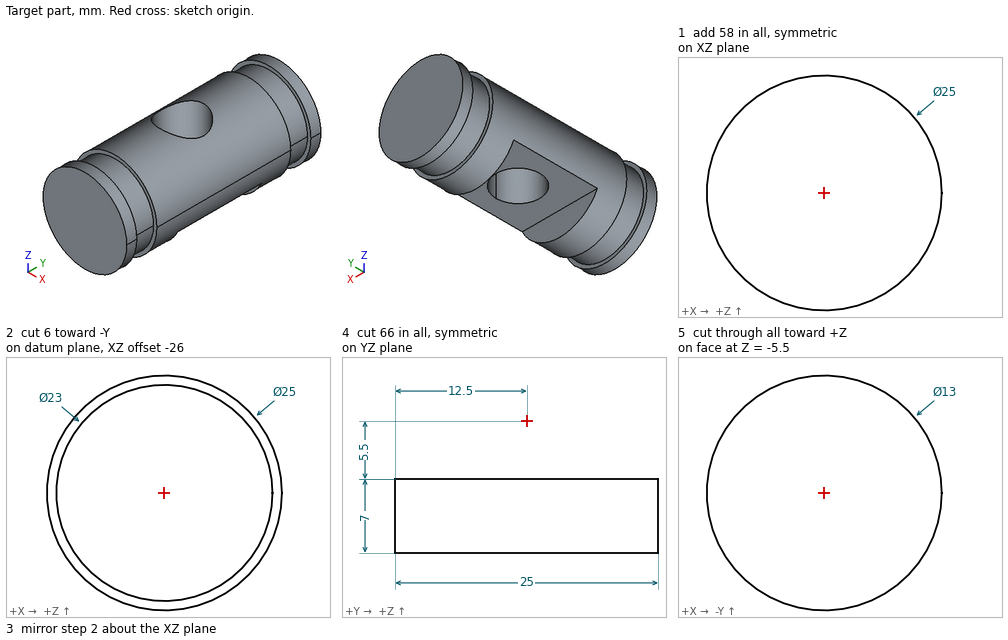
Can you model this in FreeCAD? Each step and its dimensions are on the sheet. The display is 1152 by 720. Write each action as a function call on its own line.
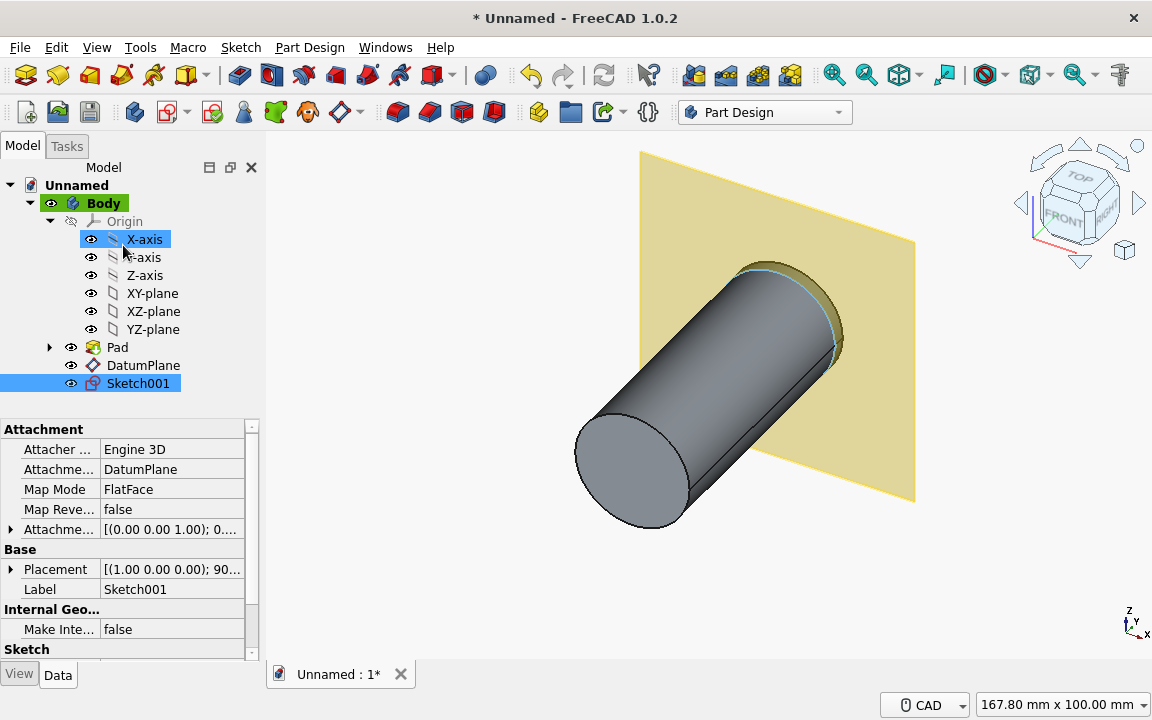
click(240, 76)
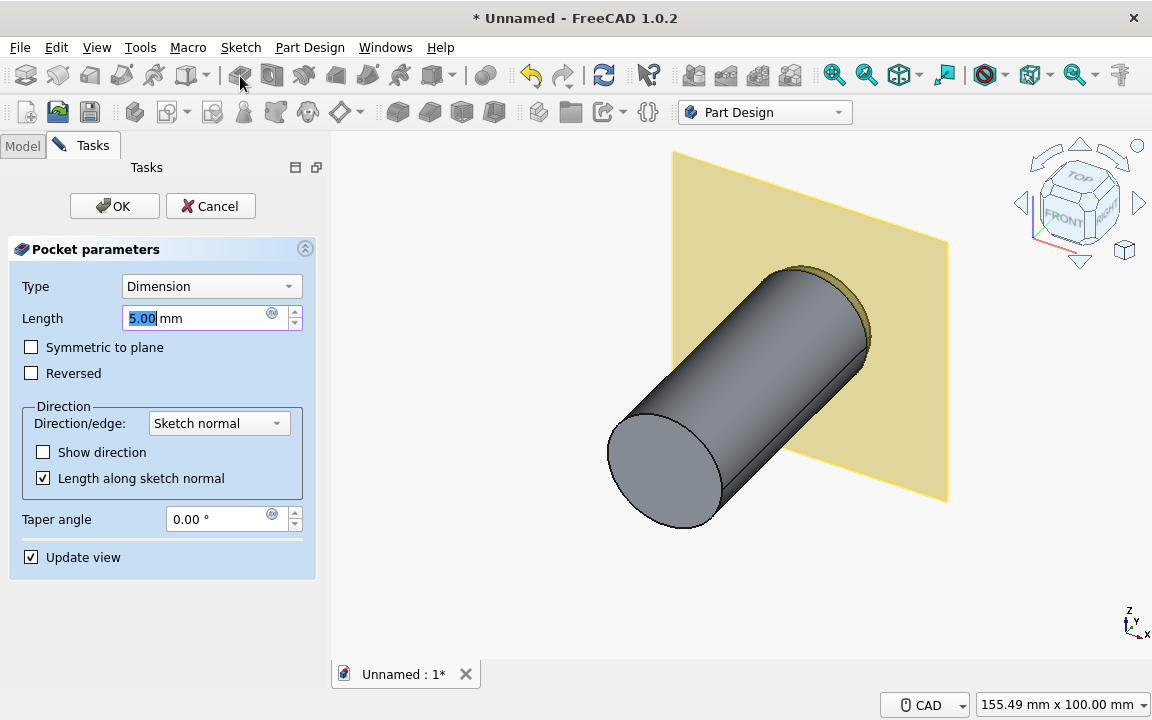
text(6)
key(Tab)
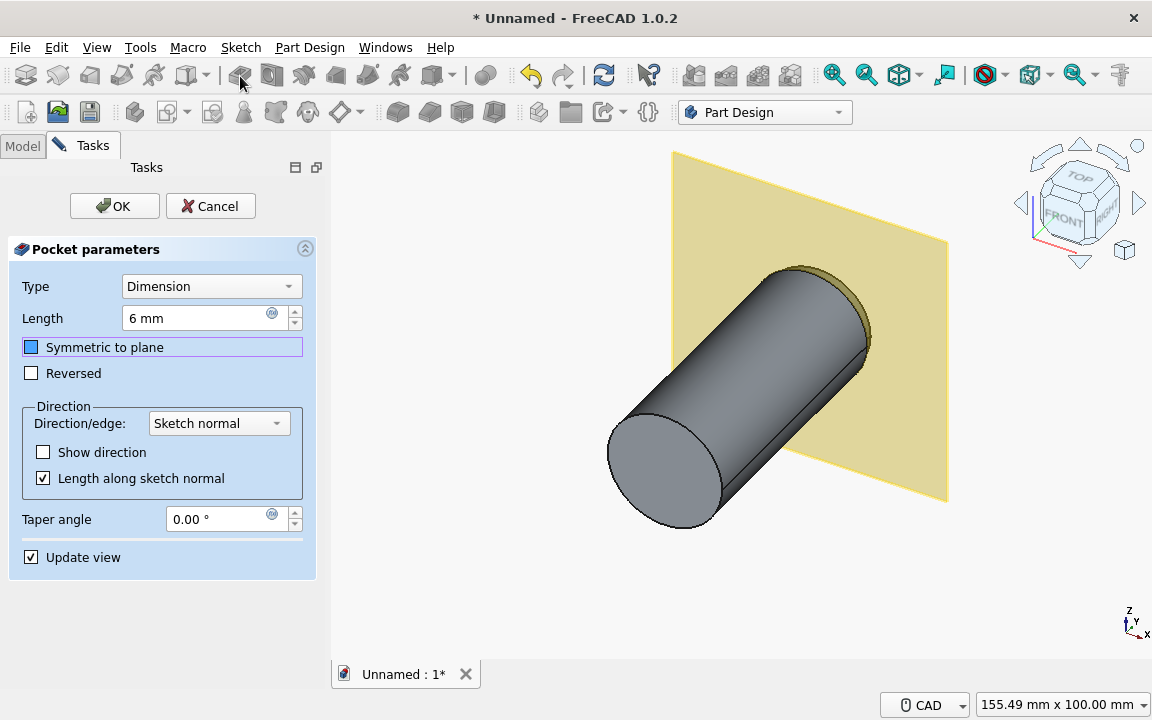
click(30, 373)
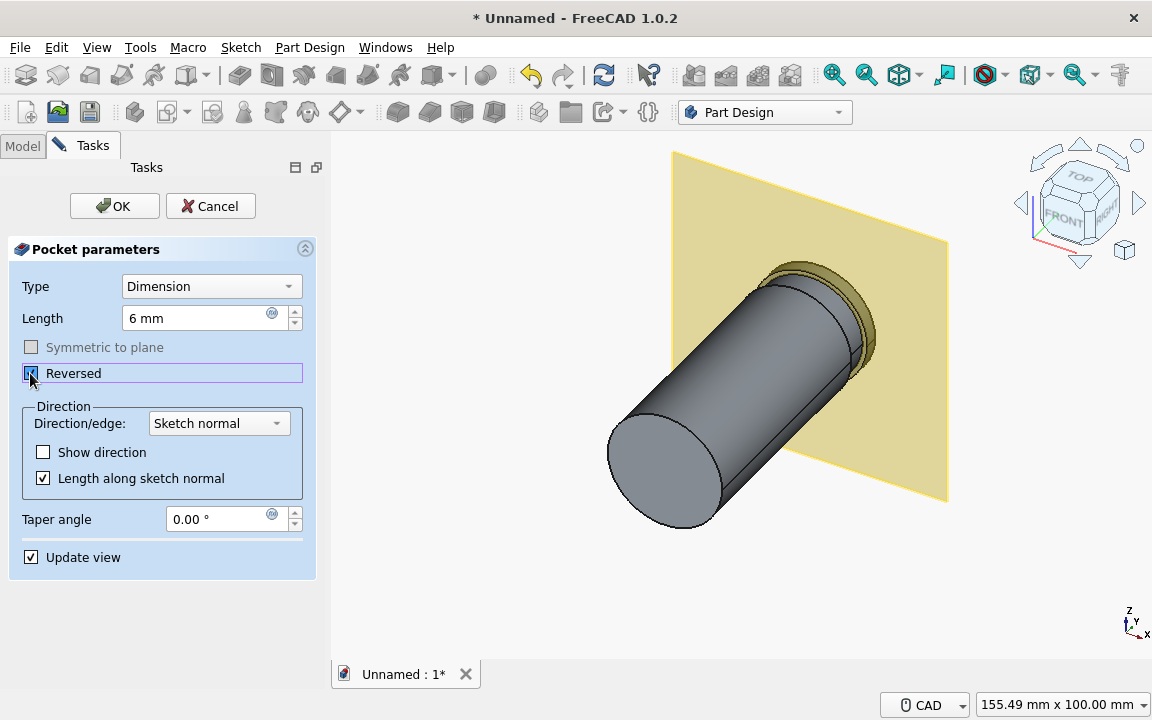
click(115, 206)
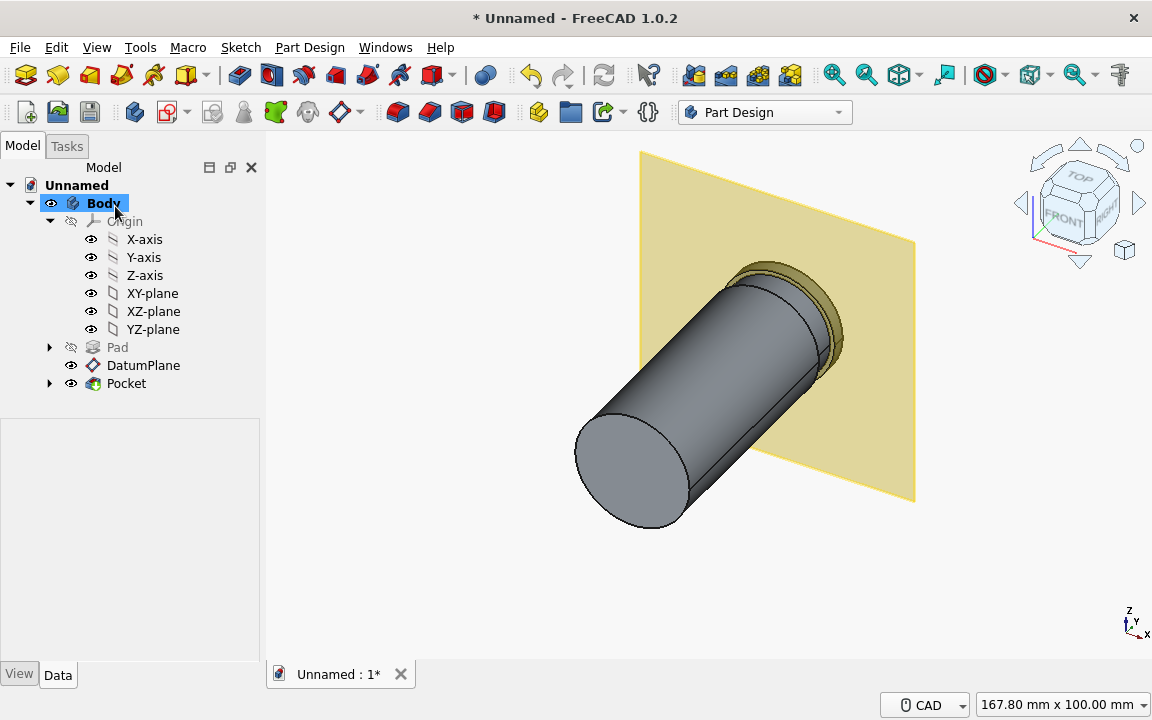
click(116, 365)
key(space)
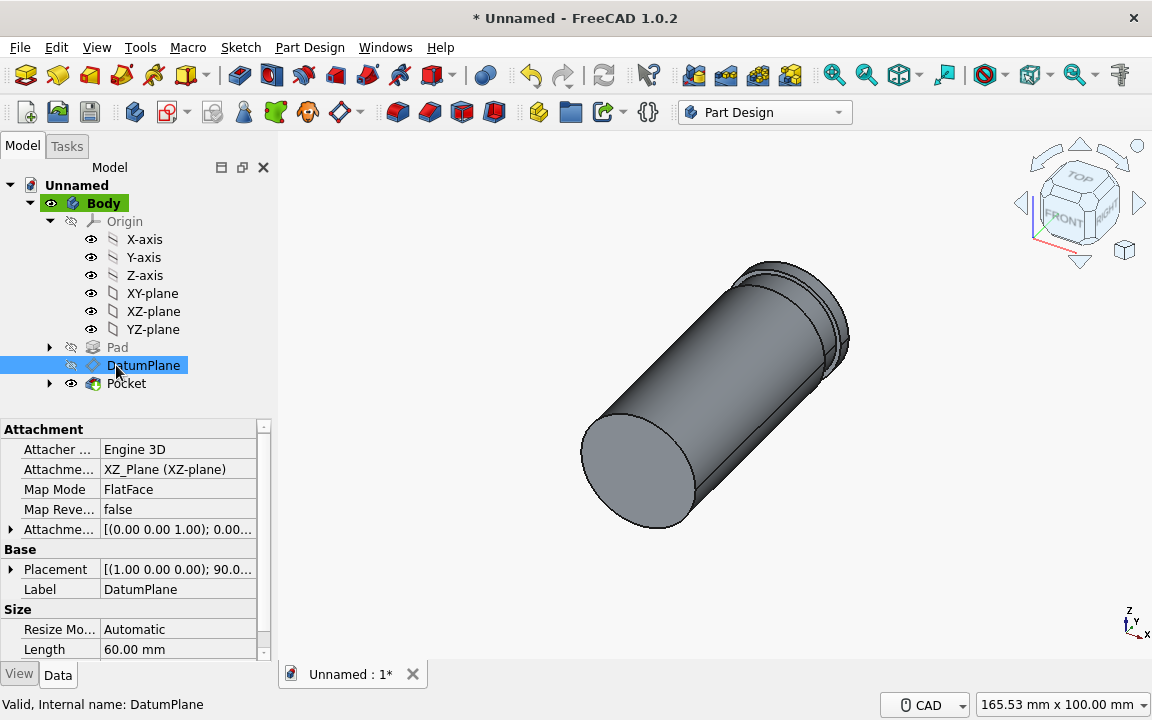
click(116, 383)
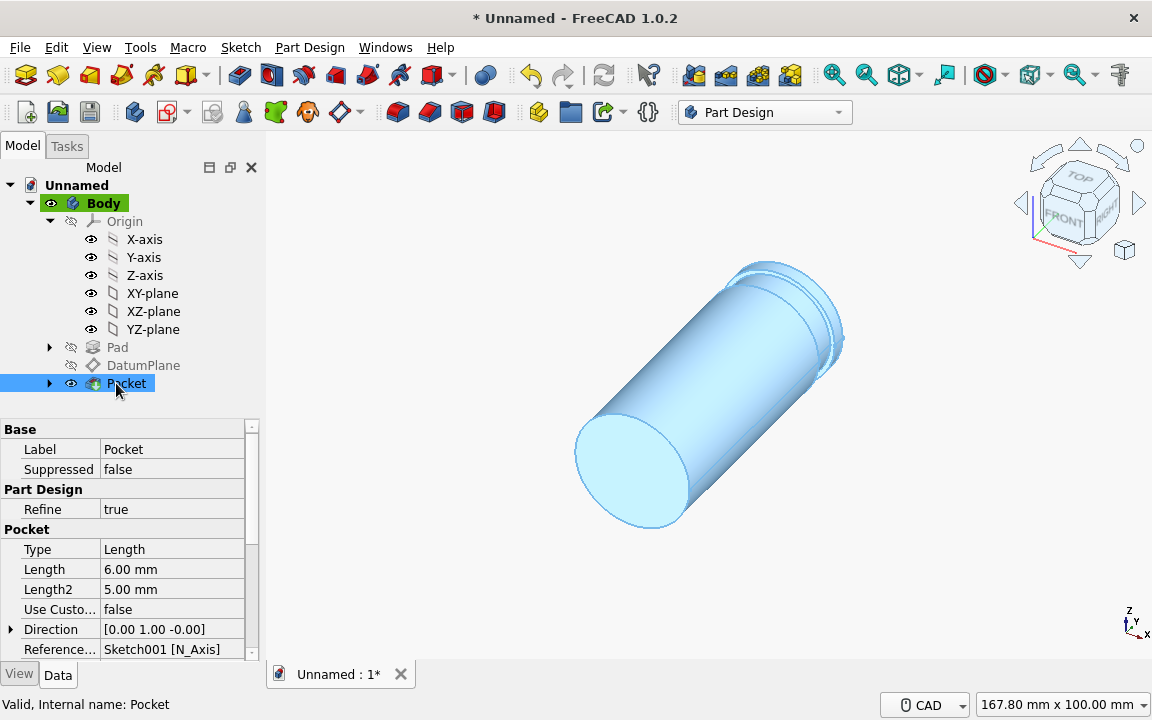
click(694, 76)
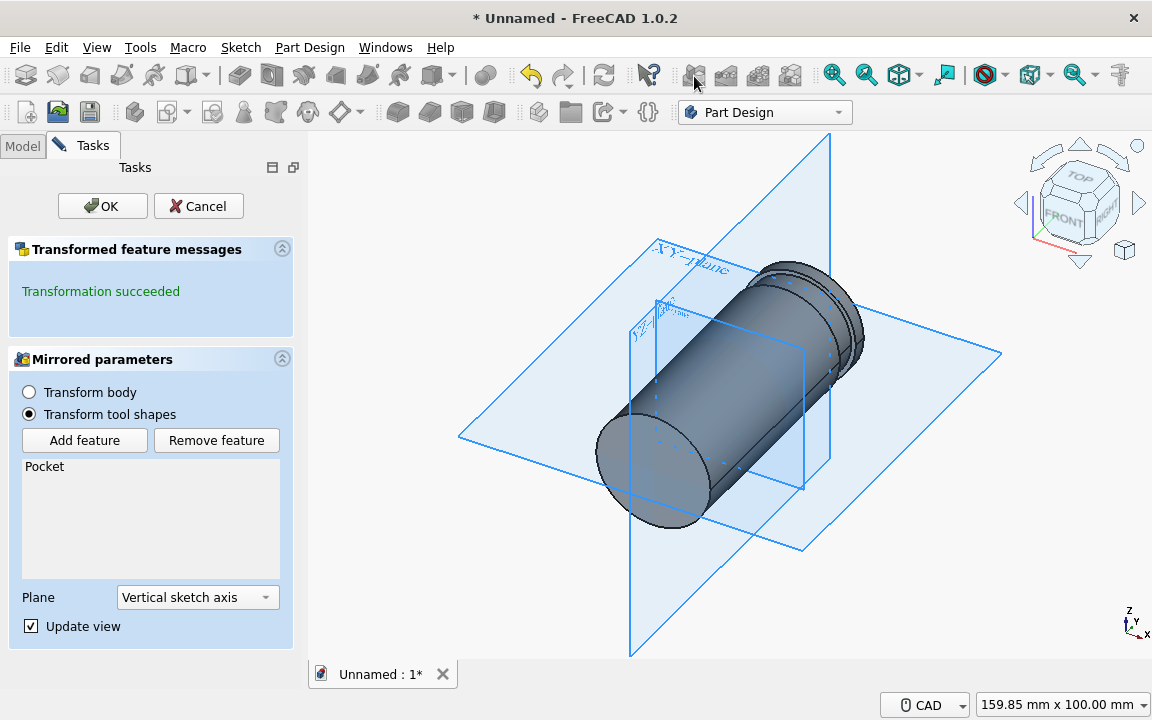
click(198, 598)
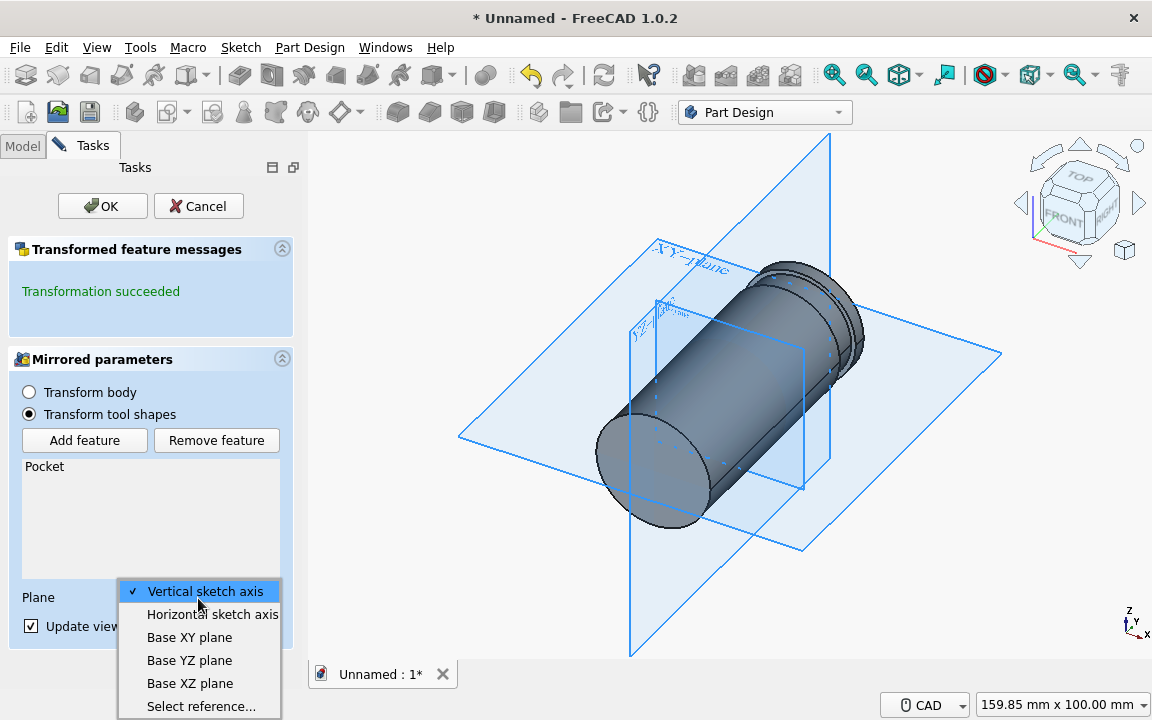
click(198, 684)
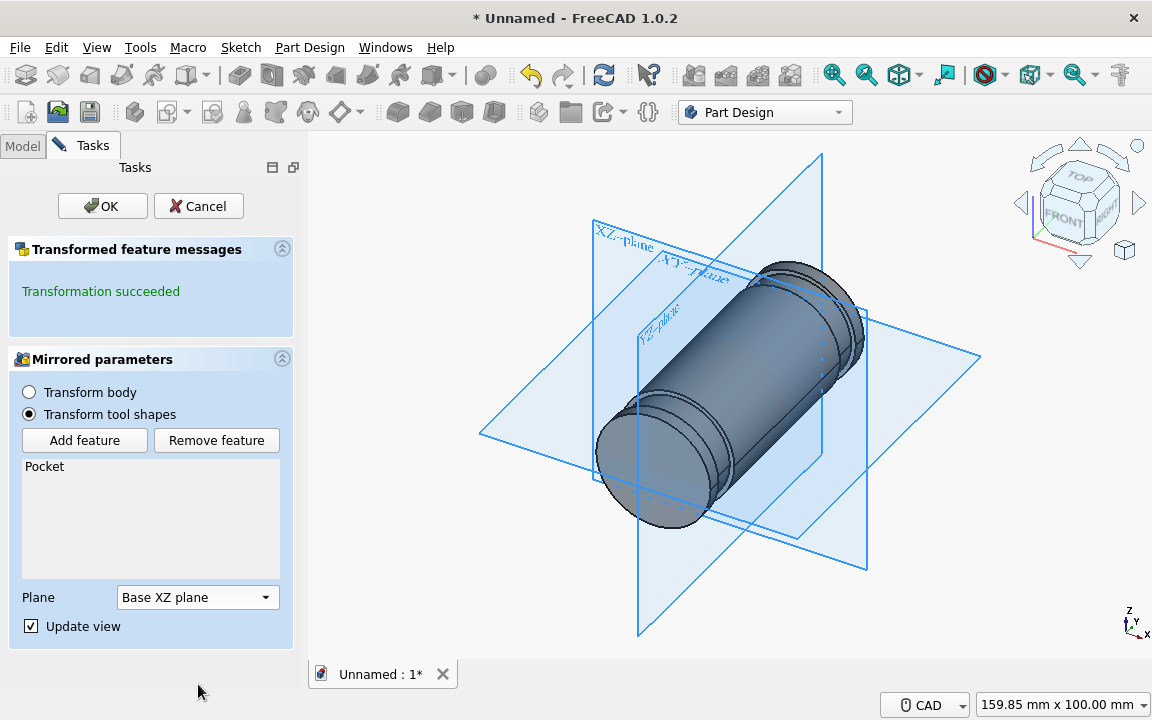
click(103, 206)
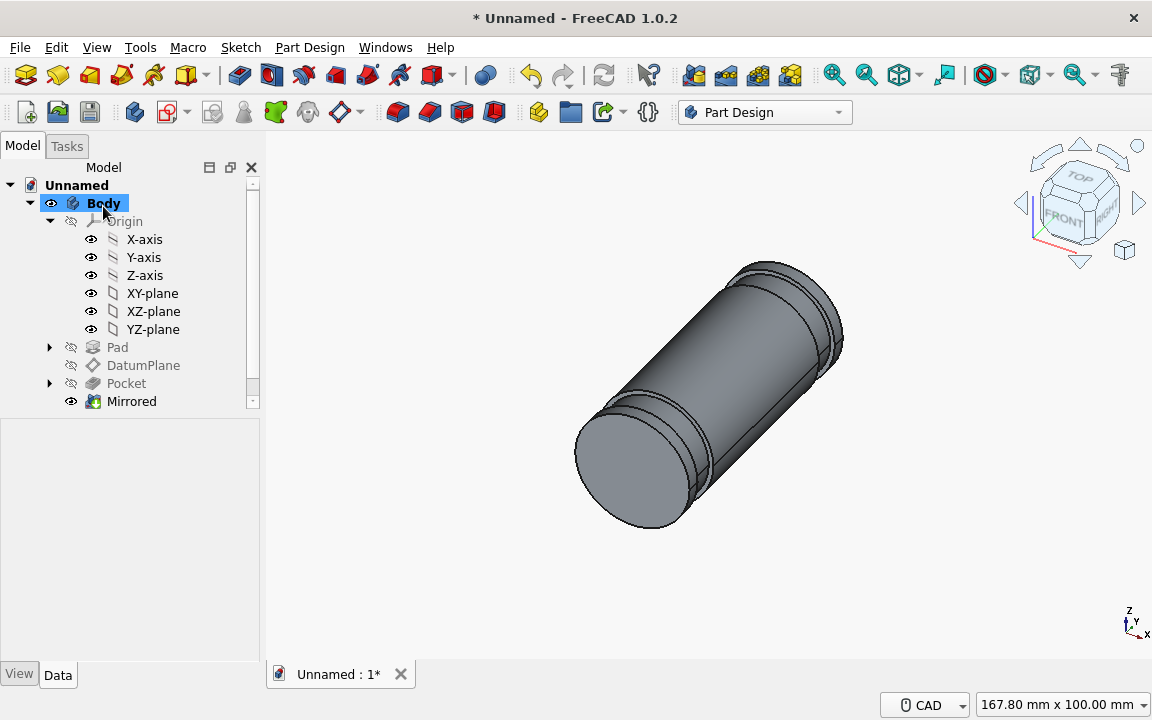
click(168, 112)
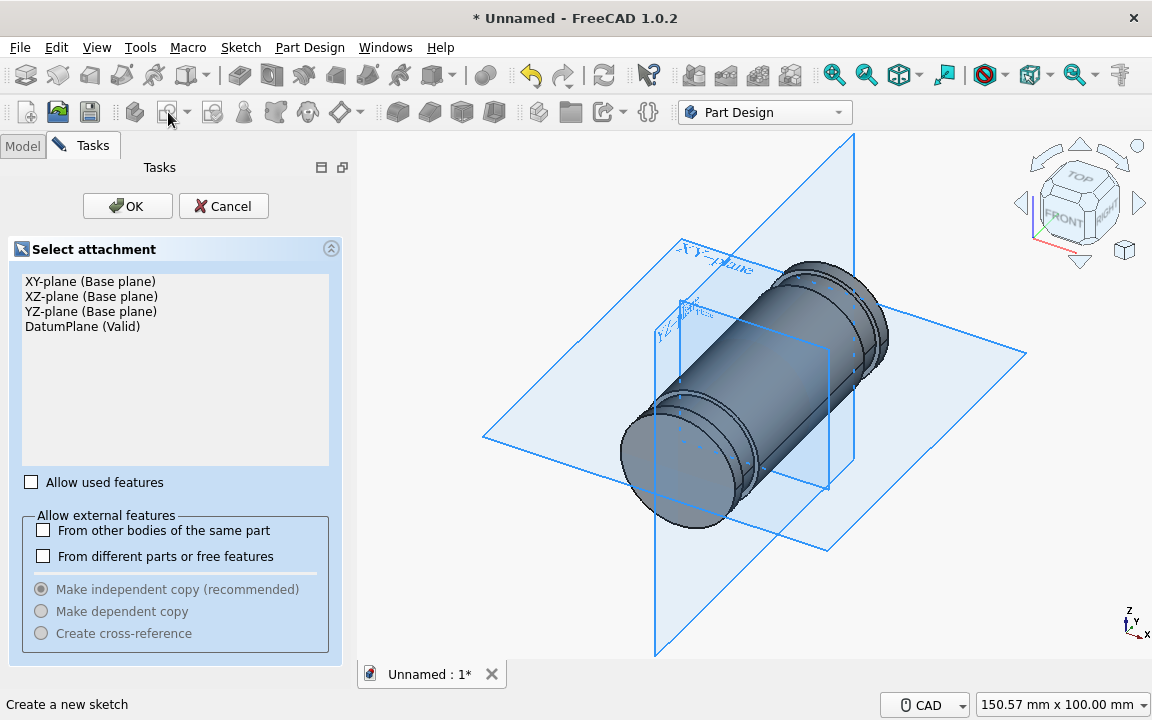
click(82, 312)